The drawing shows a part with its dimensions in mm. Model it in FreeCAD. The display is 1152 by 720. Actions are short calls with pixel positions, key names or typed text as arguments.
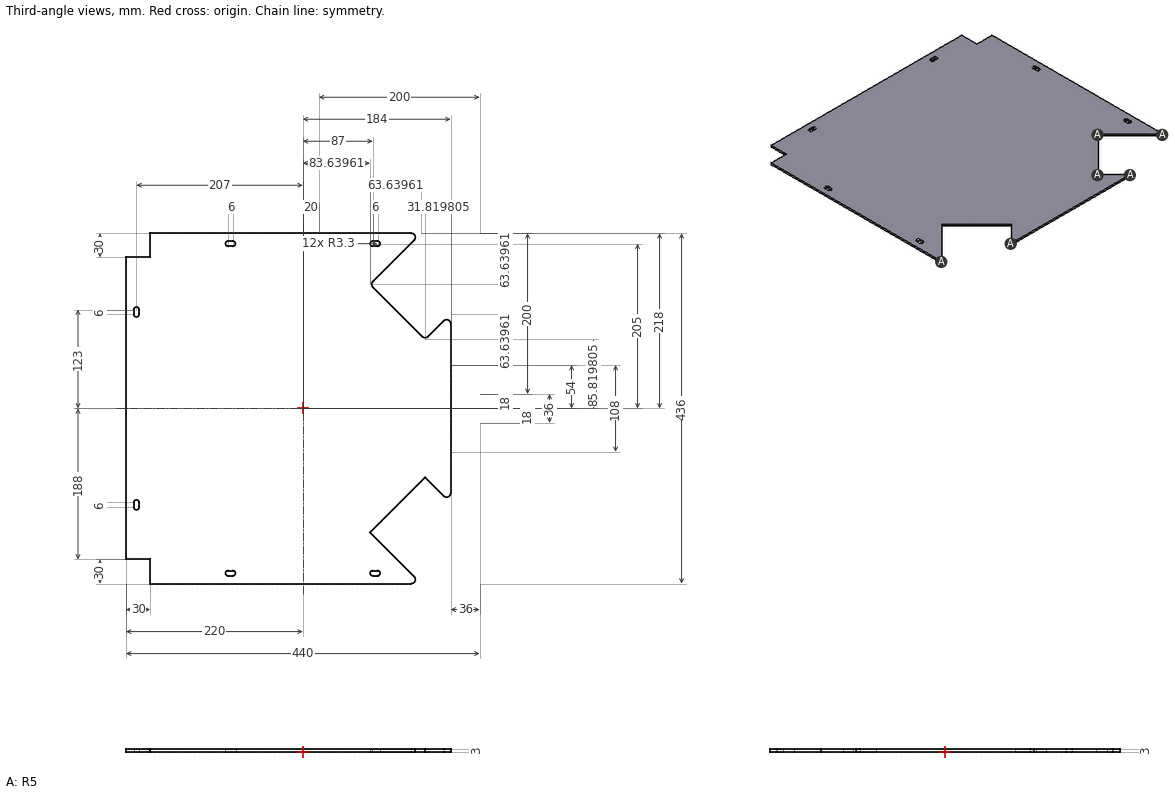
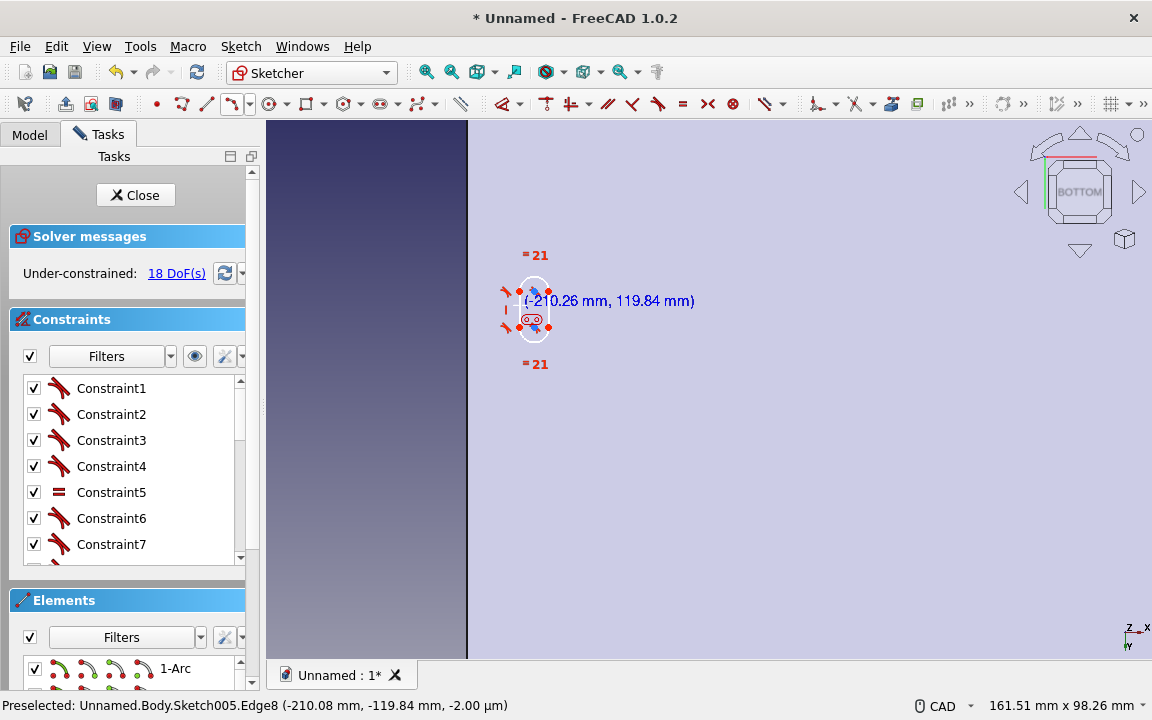
scroll(528, 300, down, 10)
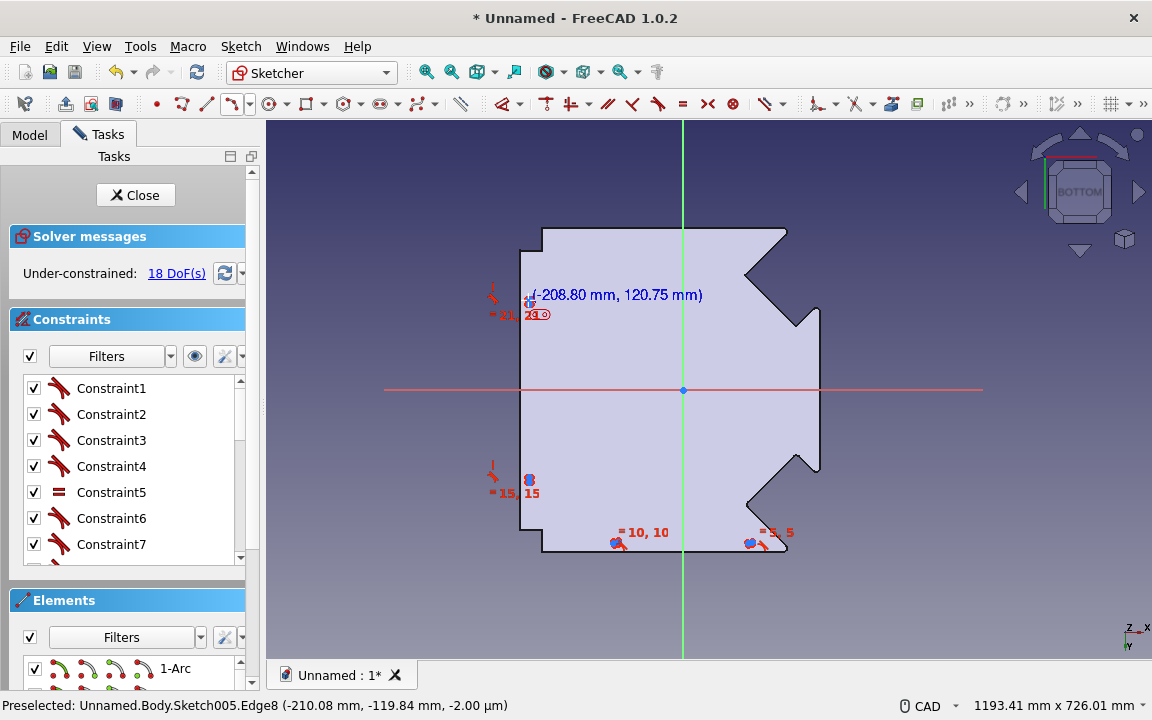
scroll(614, 238, up, 12)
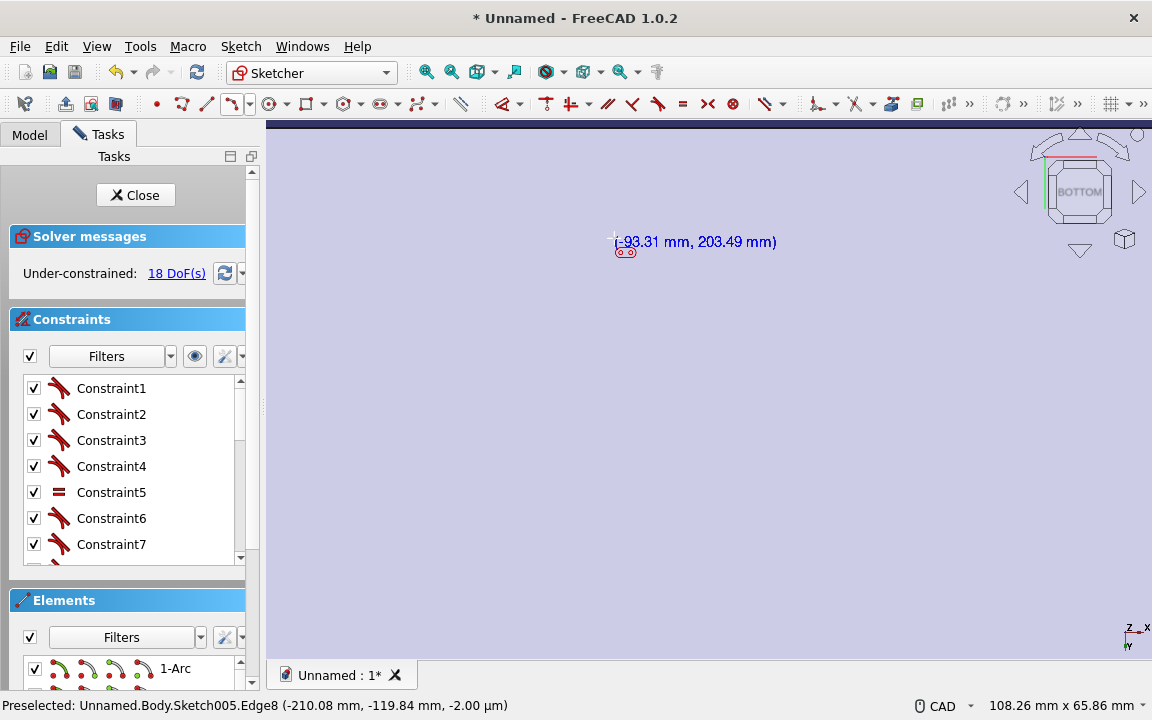
scroll(614, 238, down, 12)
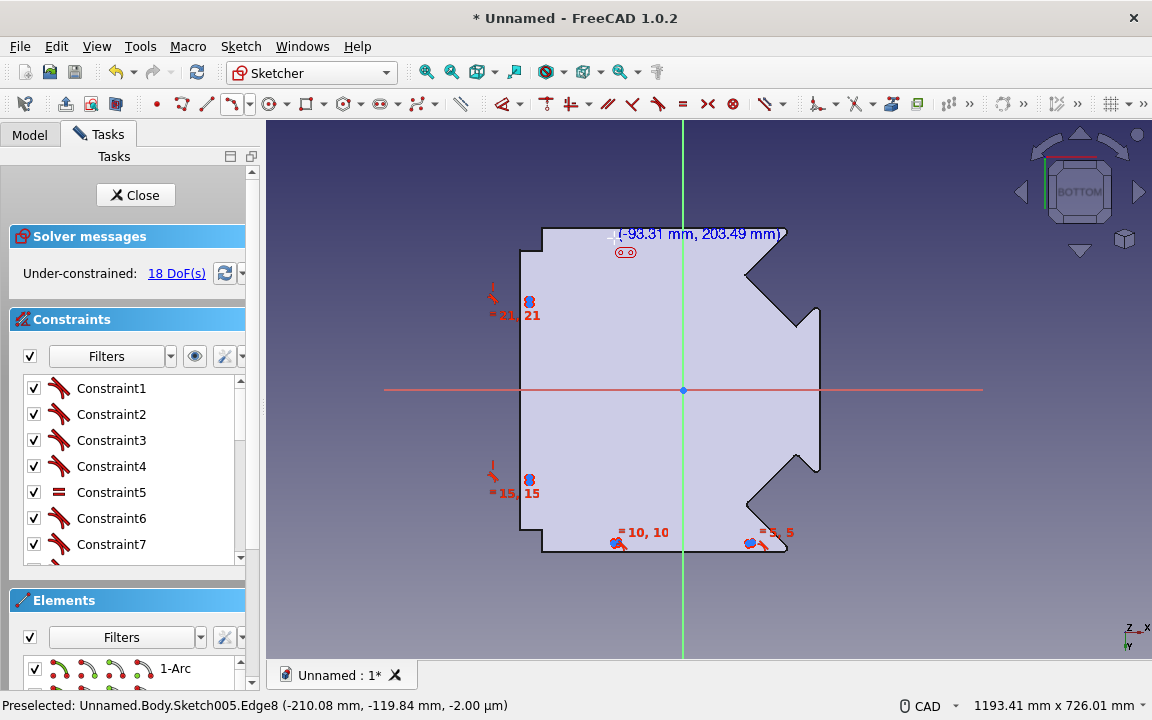
click(614, 238)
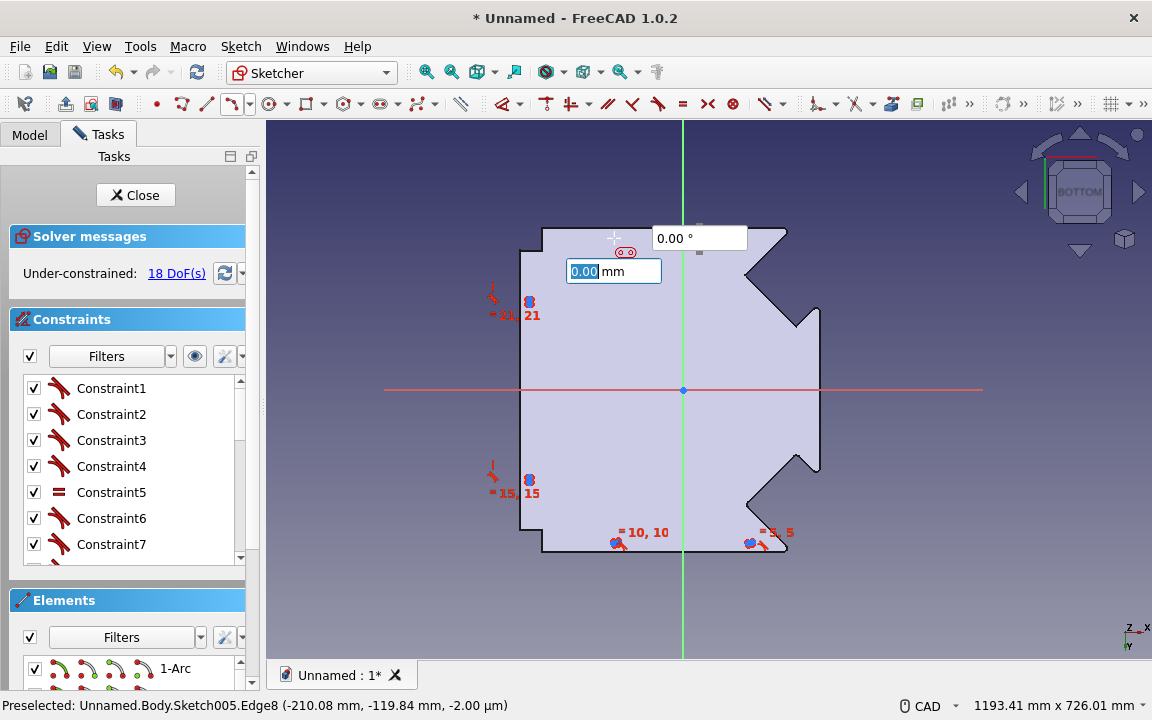
scroll(619, 238, up, 7)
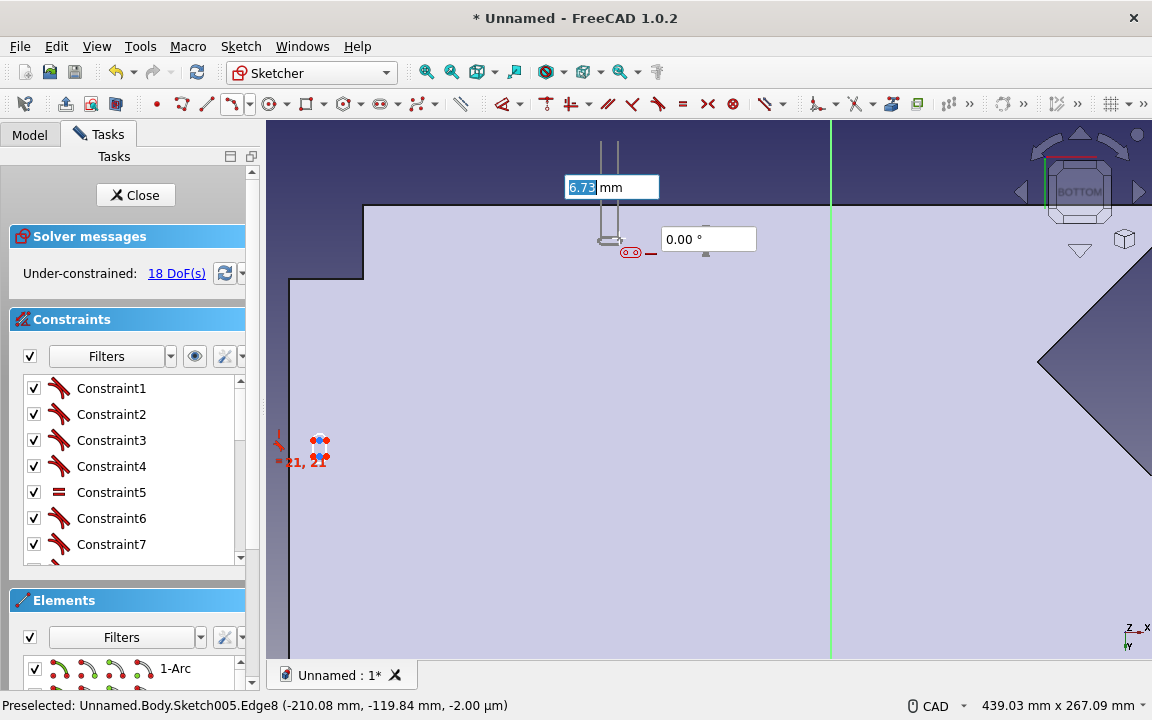
click(616, 237)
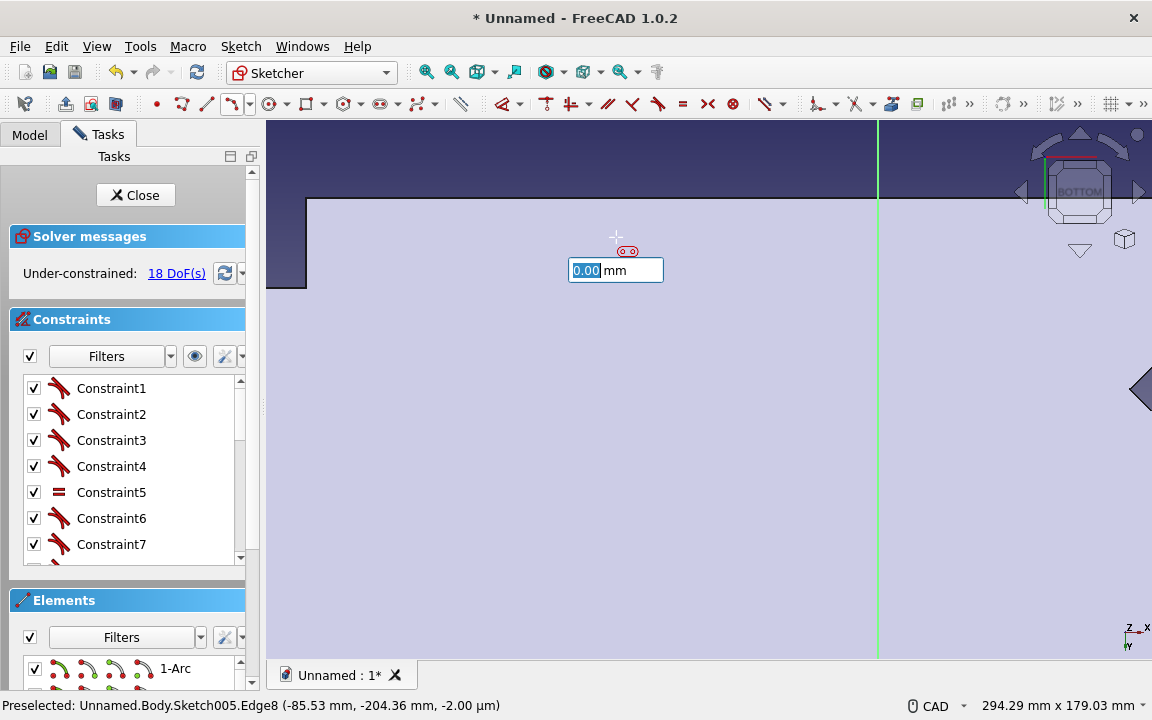
scroll(607, 227, up, 3)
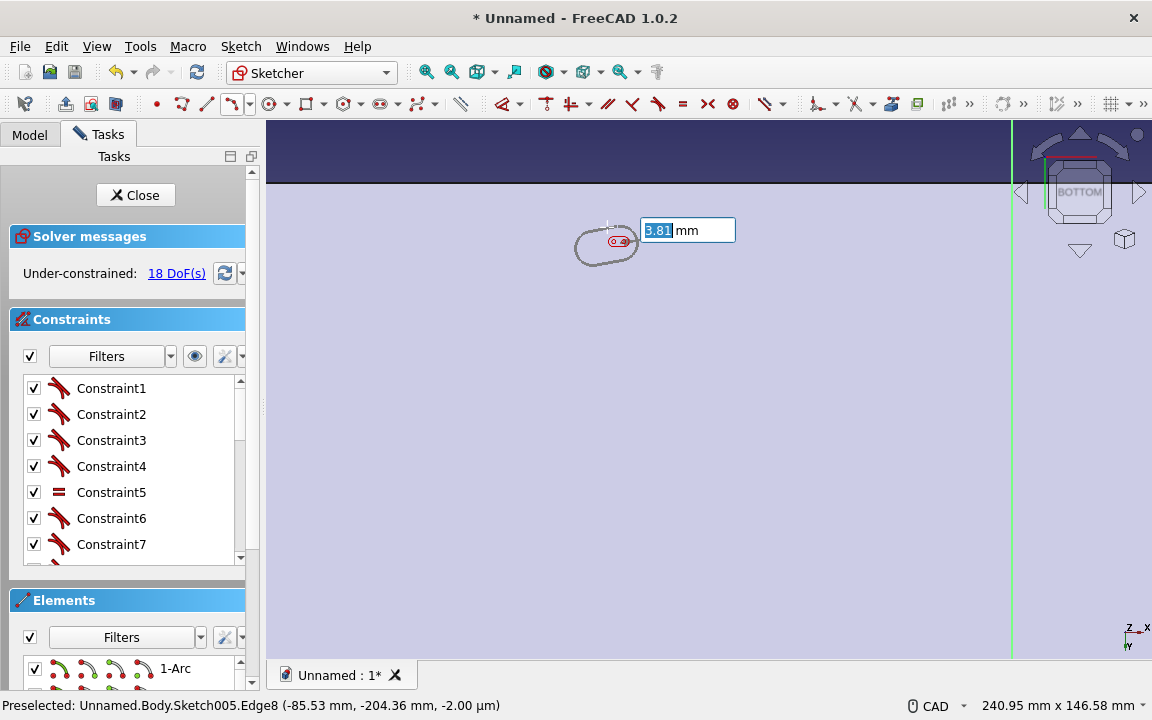
click(608, 227)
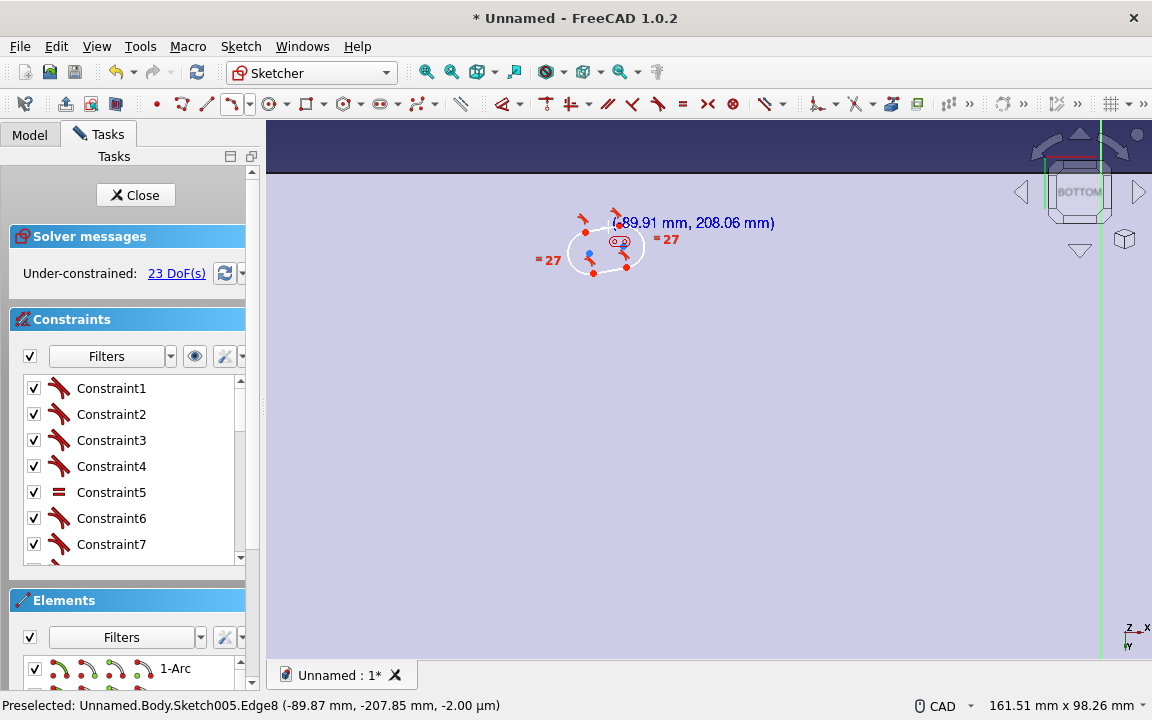
scroll(617, 236, down, 10)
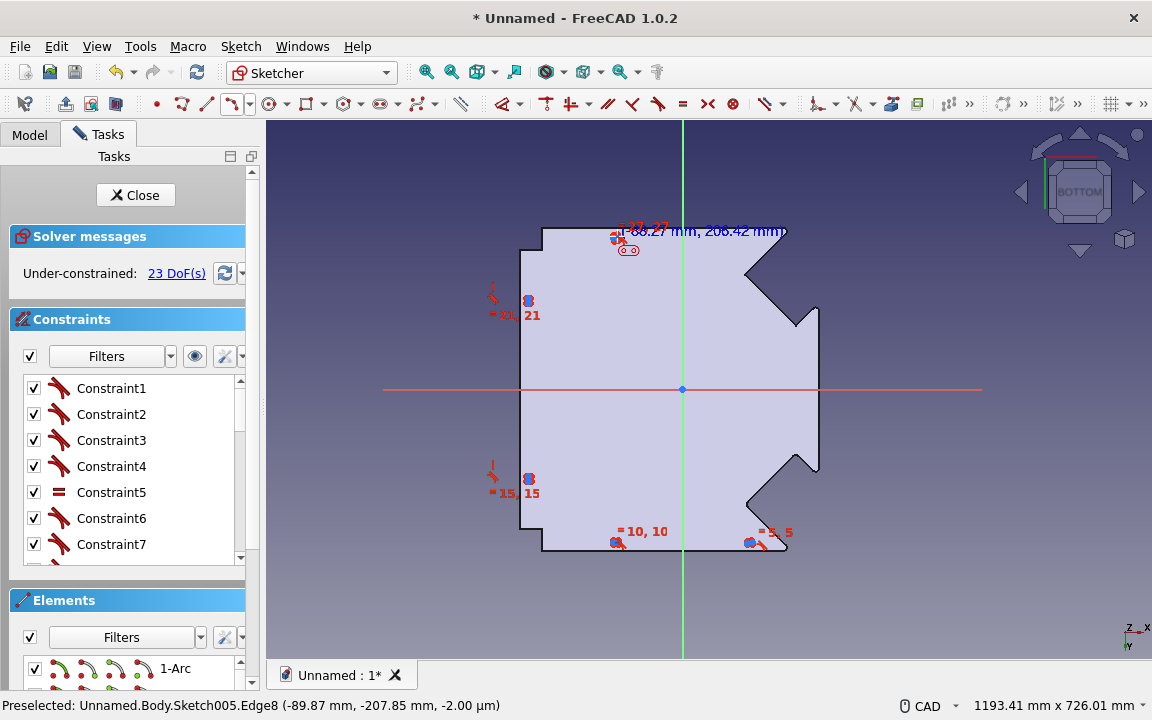
scroll(747, 237, up, 12)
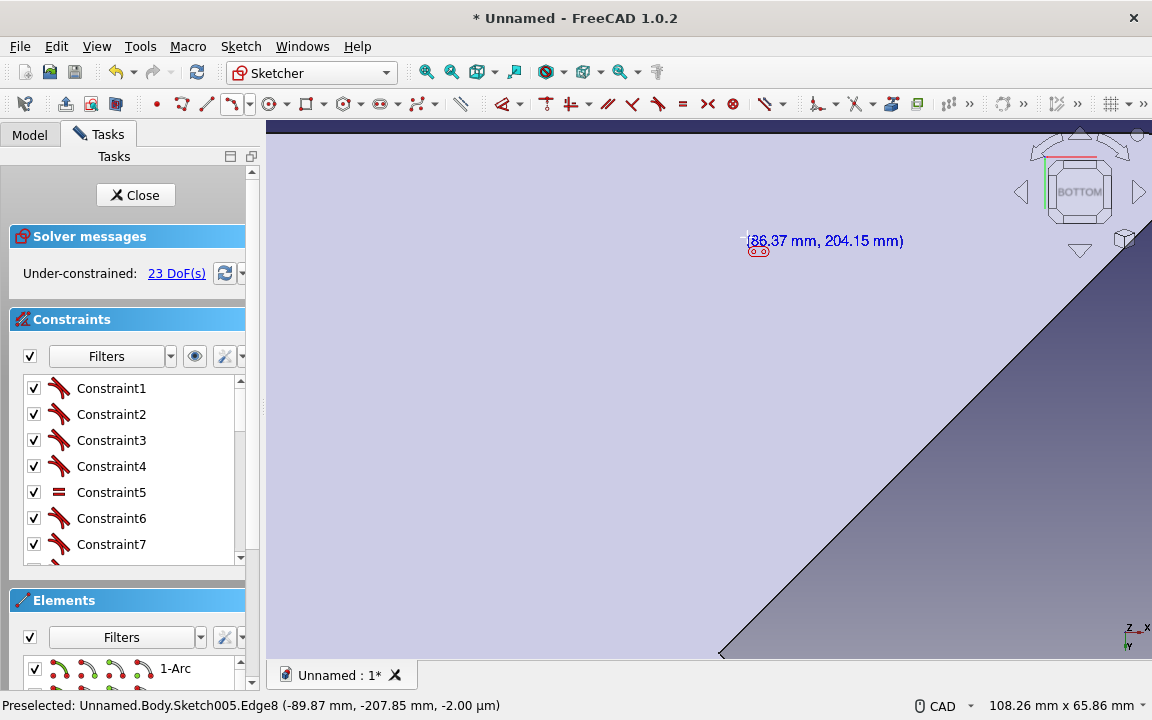
scroll(747, 237, down, 12)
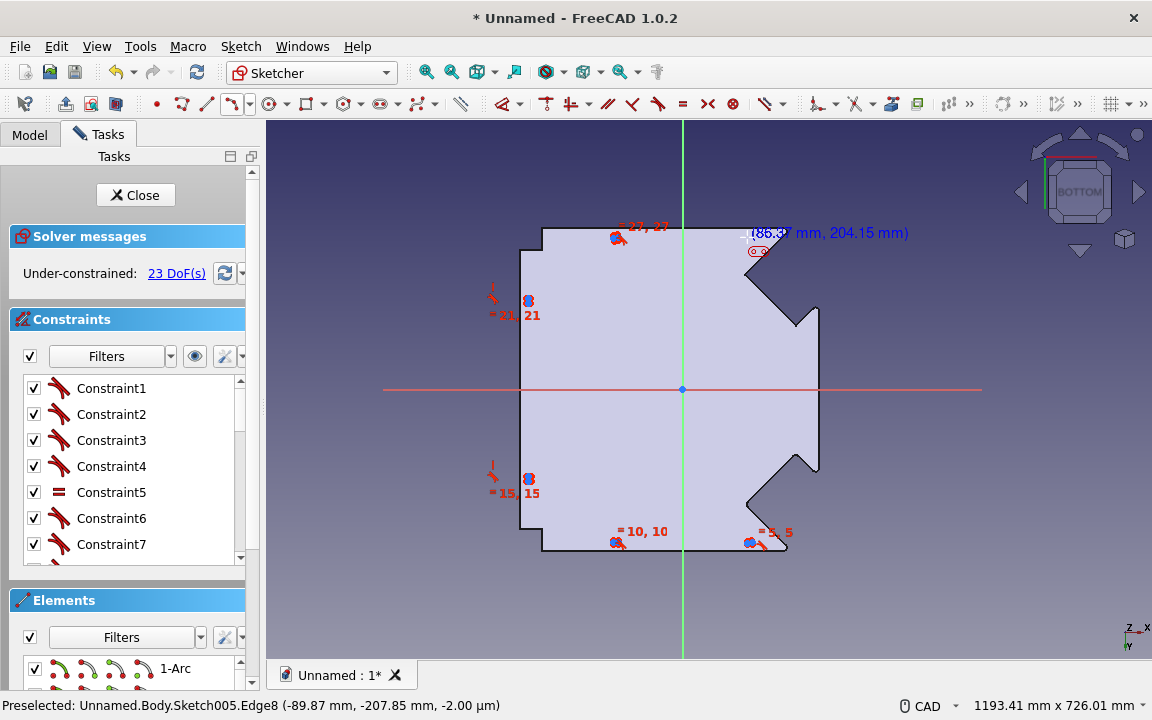
click(747, 237)